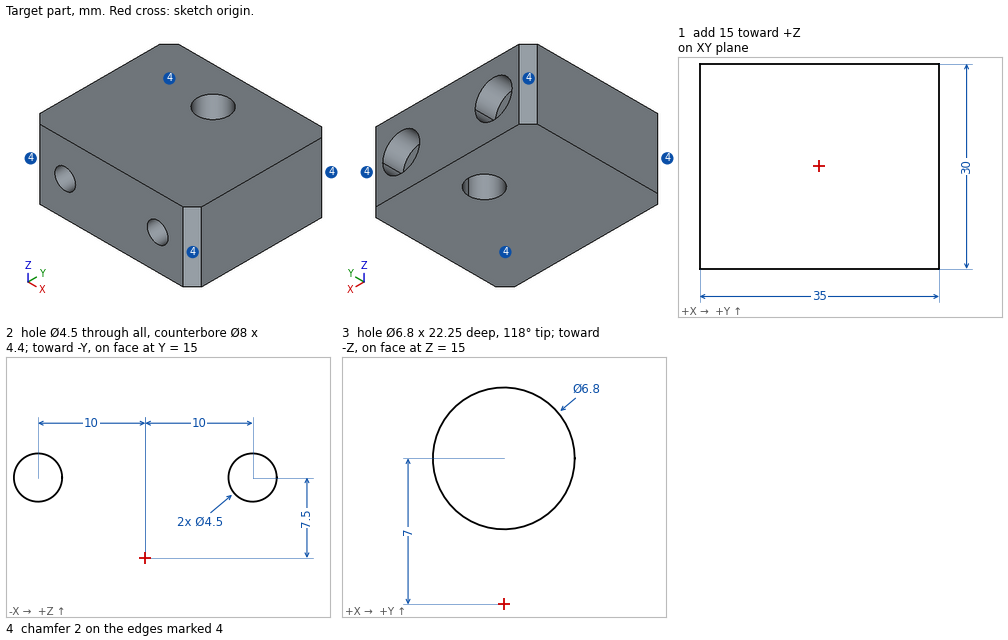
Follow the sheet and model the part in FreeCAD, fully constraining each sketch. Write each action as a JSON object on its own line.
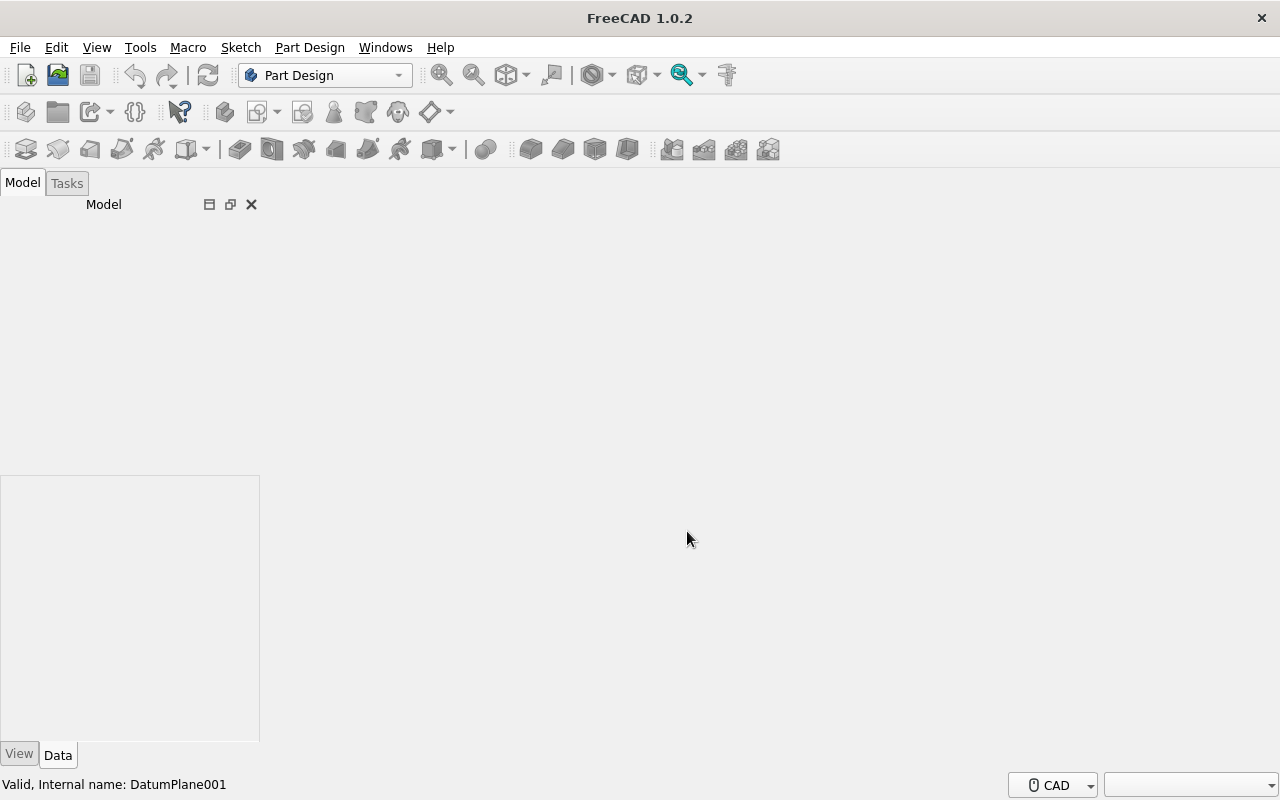
{"action": "key", "text": "ctrl+n"}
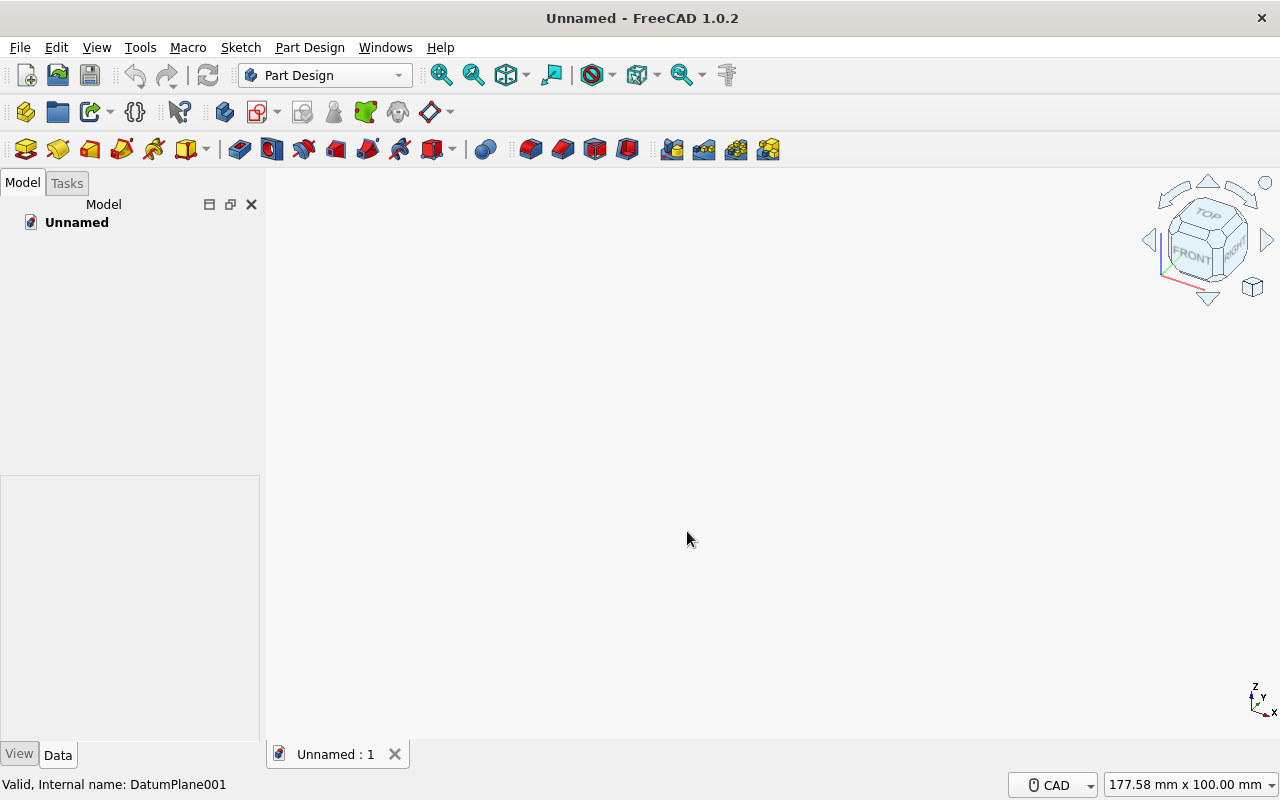
{"action": "left_click", "coordinate": [258, 112]}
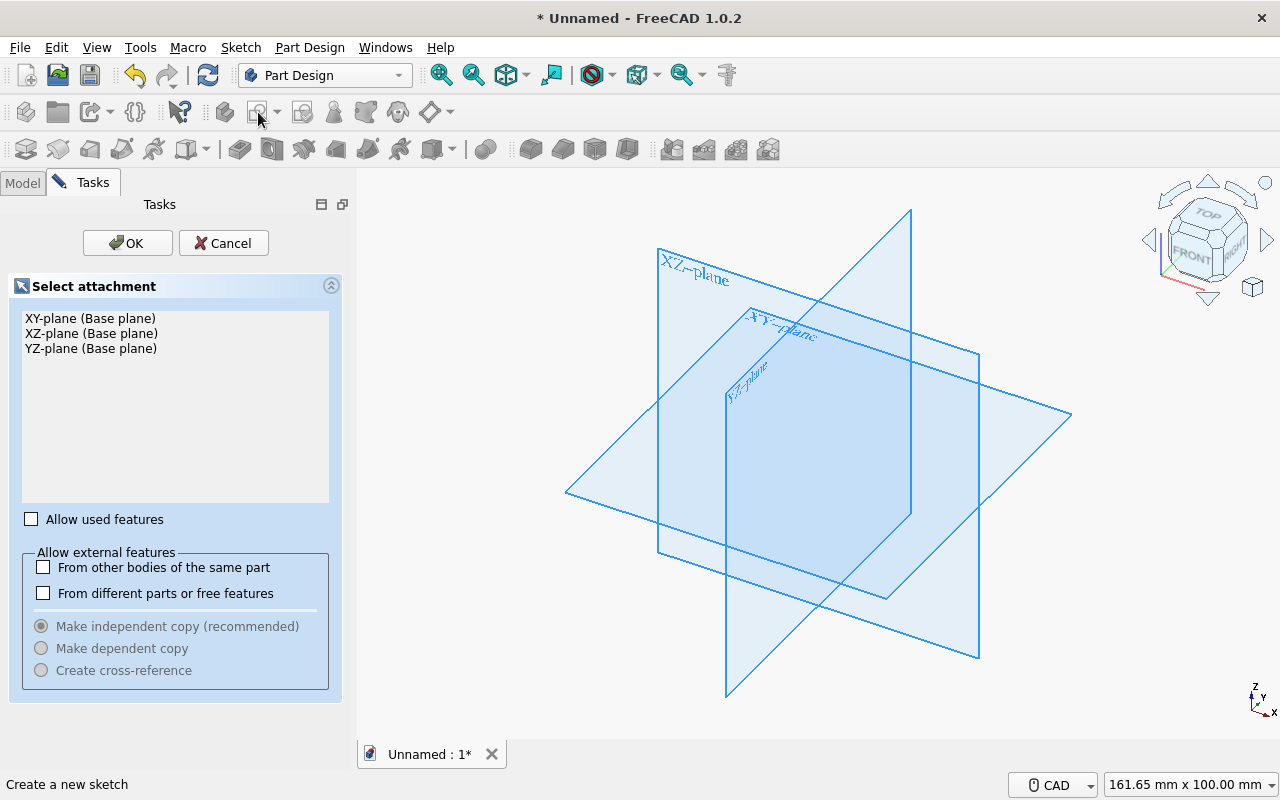
{"action": "left_click", "coordinate": [82, 318]}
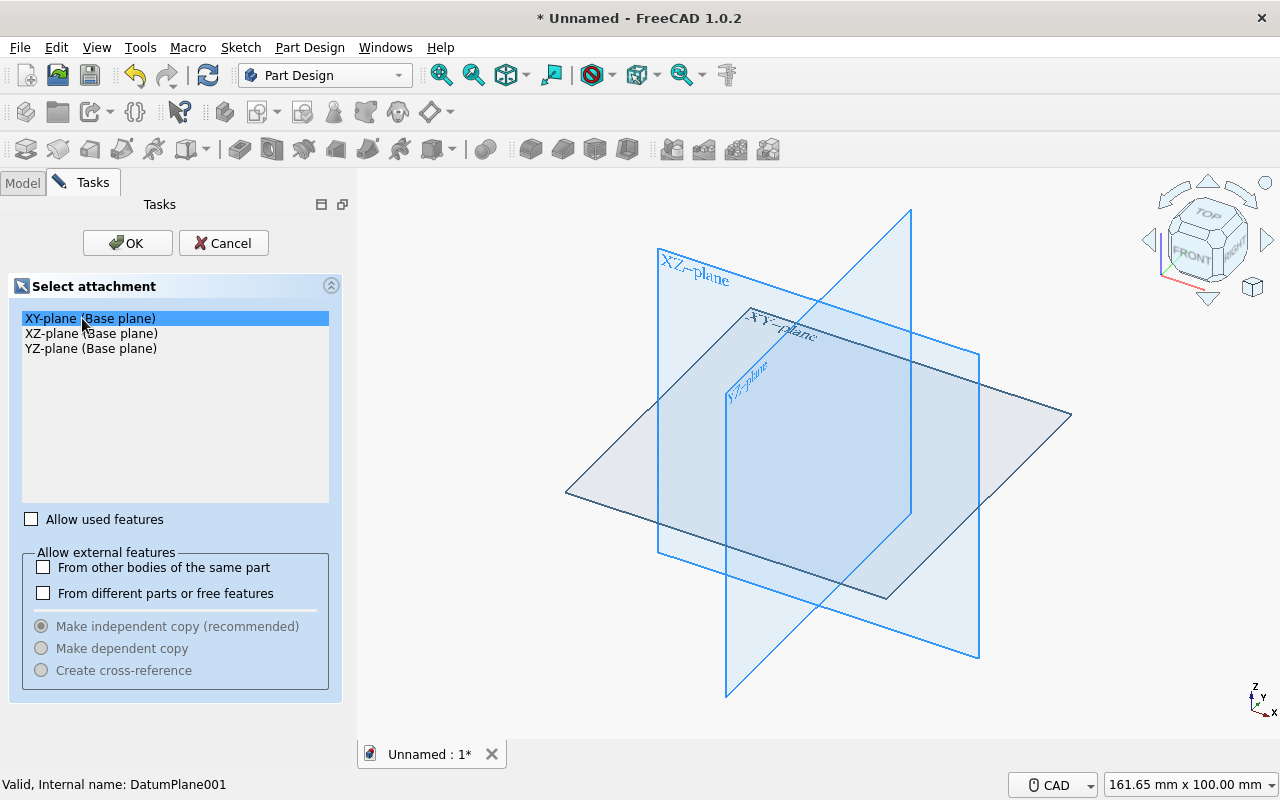
{"action": "left_click", "coordinate": [128, 243]}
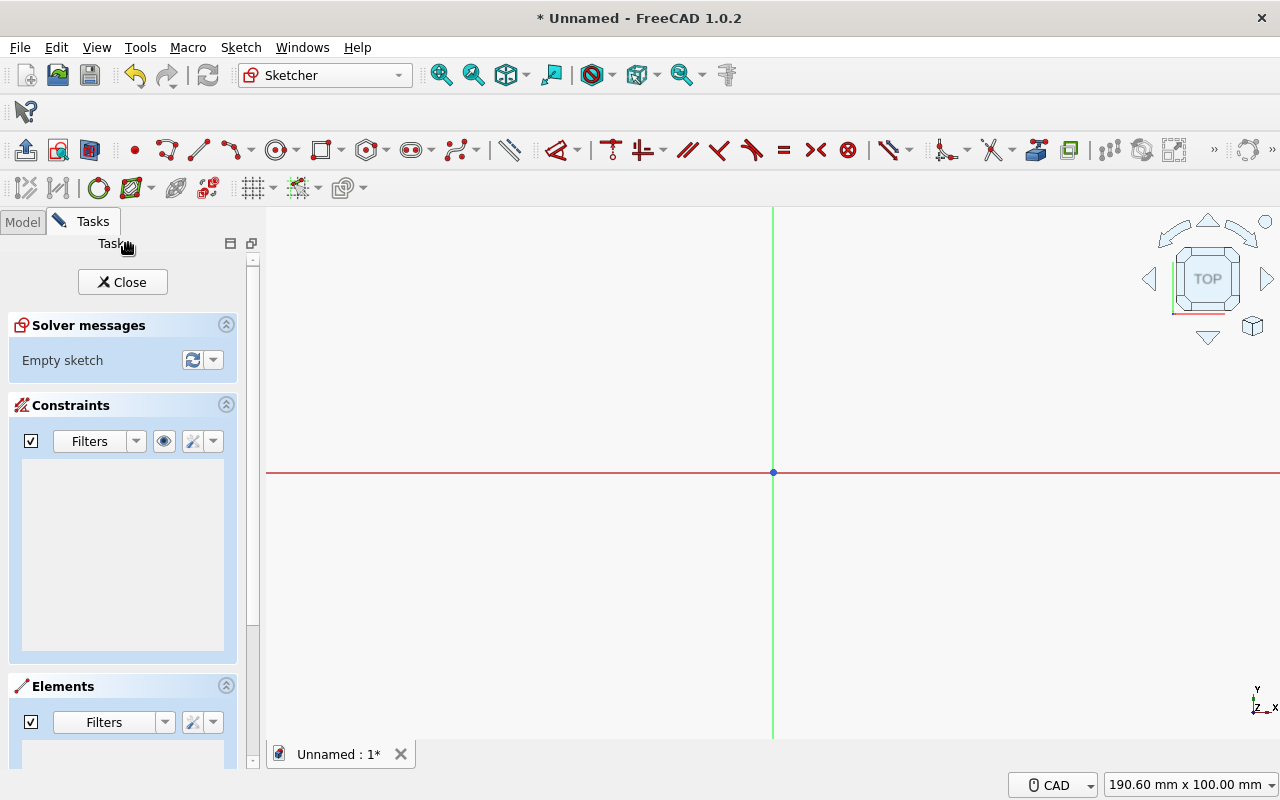
{"action": "scroll", "coordinate": [829, 473], "scroll_direction": "up", "scroll_amount": 4}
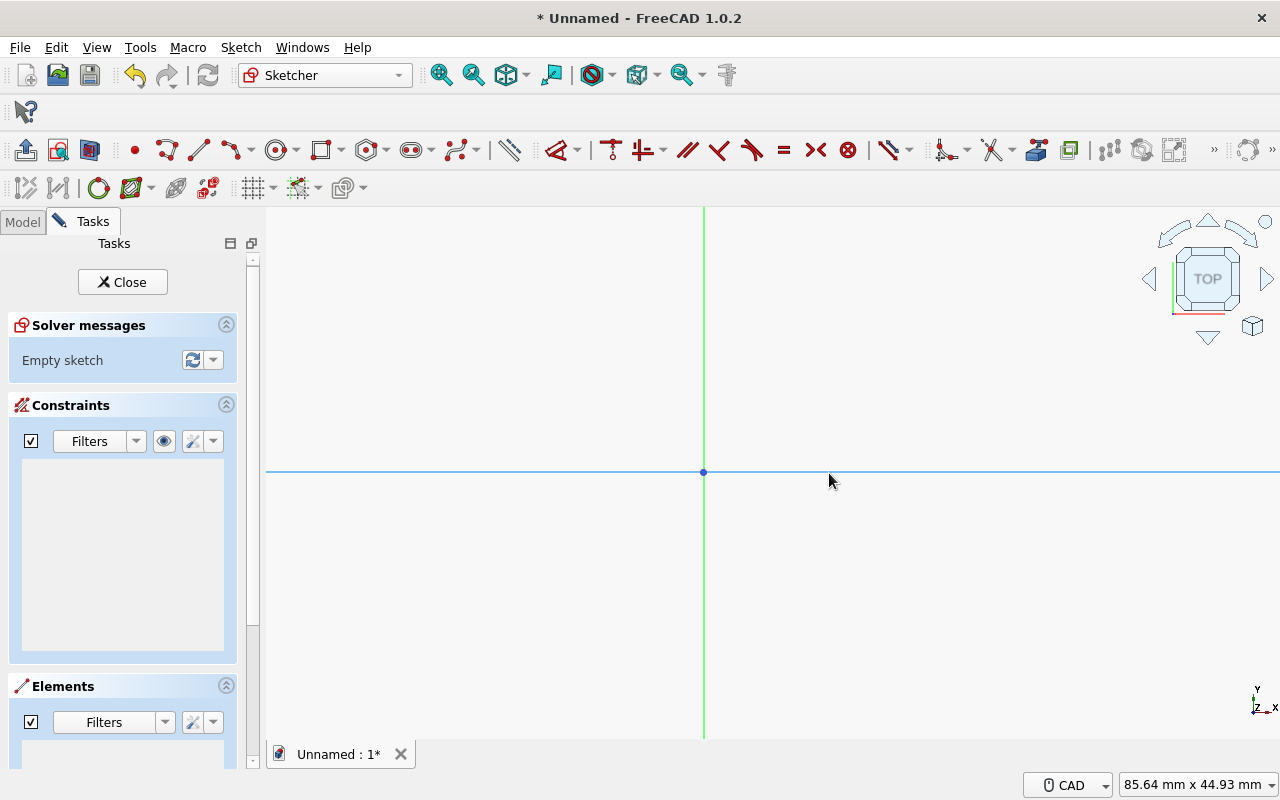
{"action": "key", "text": "g v"}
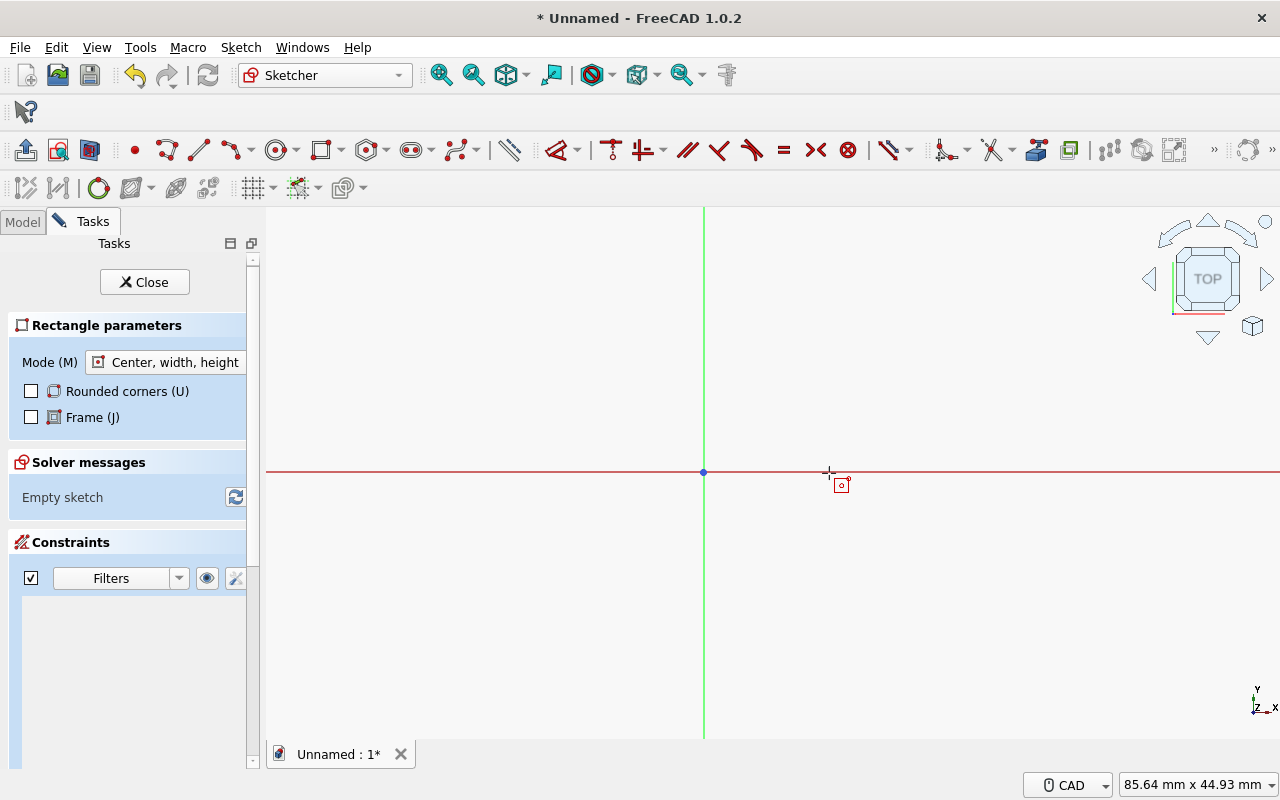
{"action": "left_click", "coordinate": [704, 472]}
{"action": "mouse_move", "coordinate": [911, 295]}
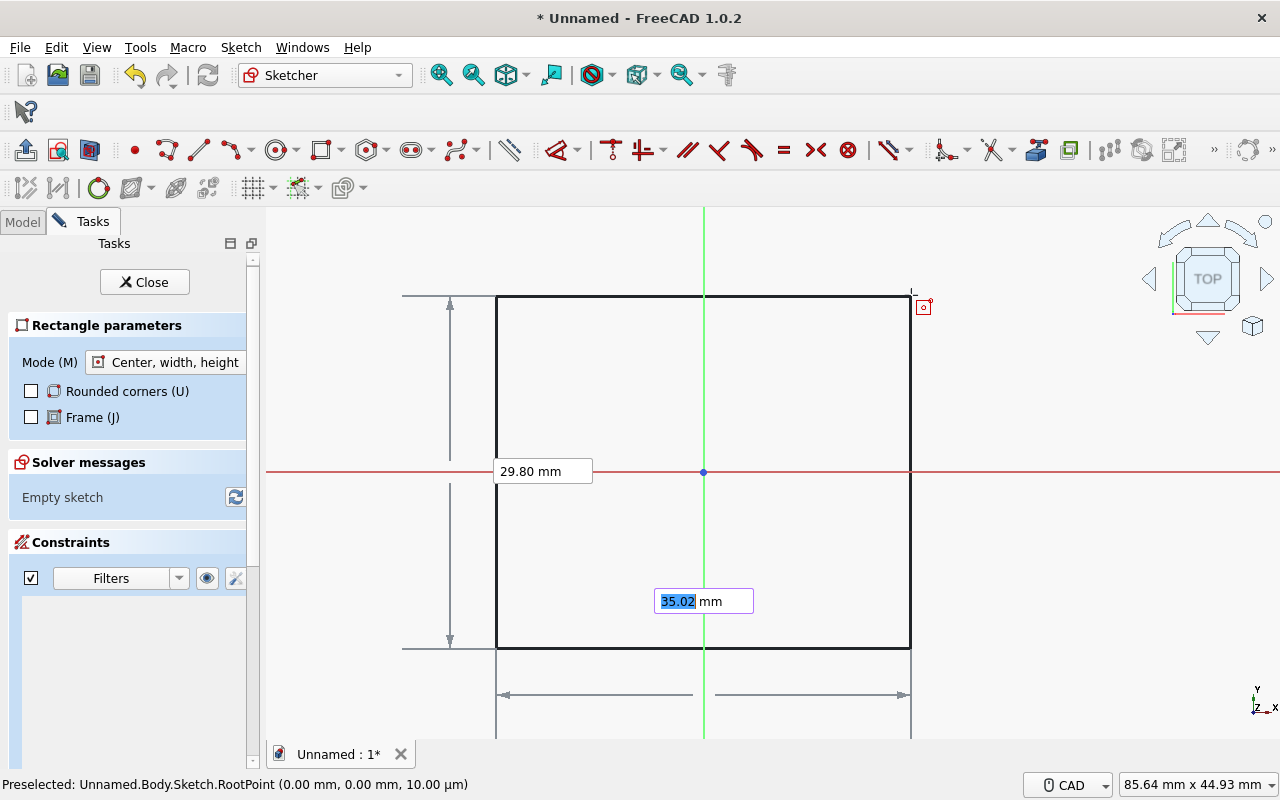
{"action": "type", "text": "35"}
{"action": "key", "text": "Tab"}
{"action": "type", "text": "30"}
{"action": "key", "text": "Return"}
{"action": "key", "text": "Escape"}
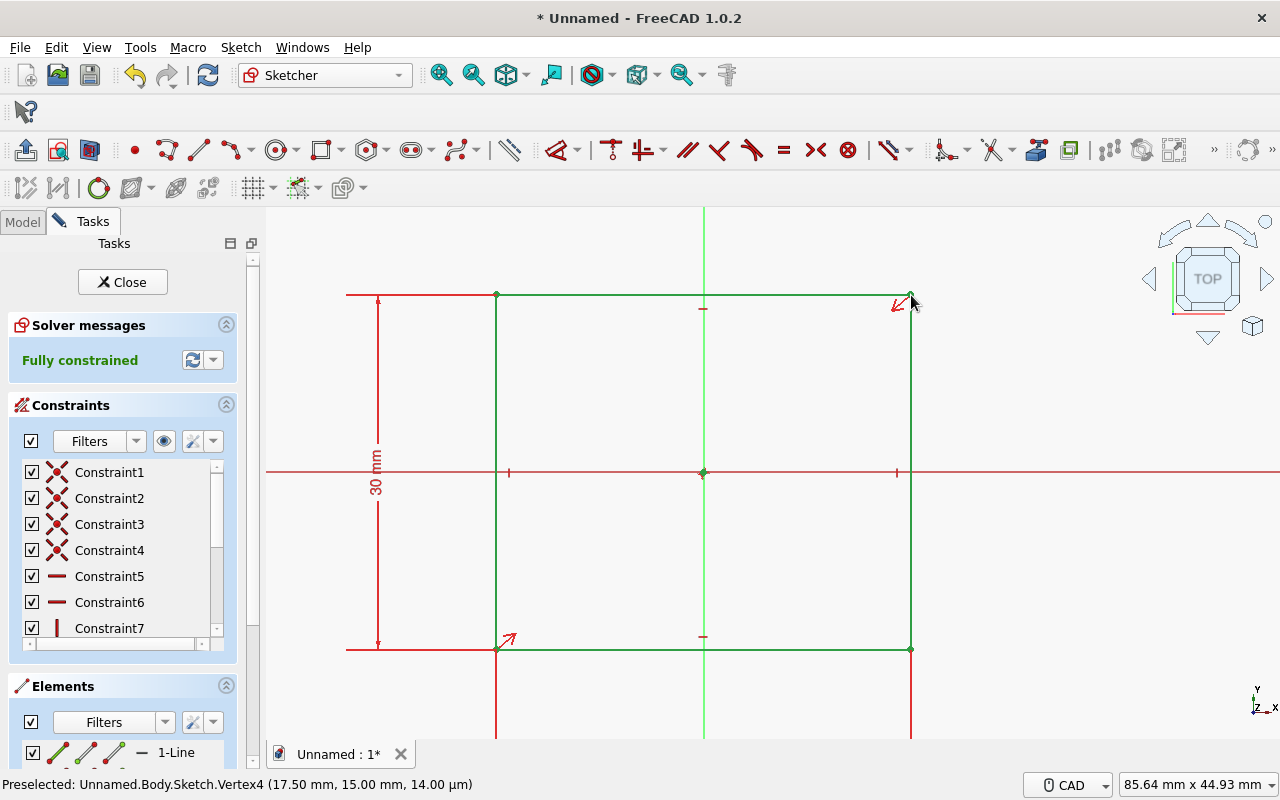
{"action": "left_click", "coordinate": [123, 282]}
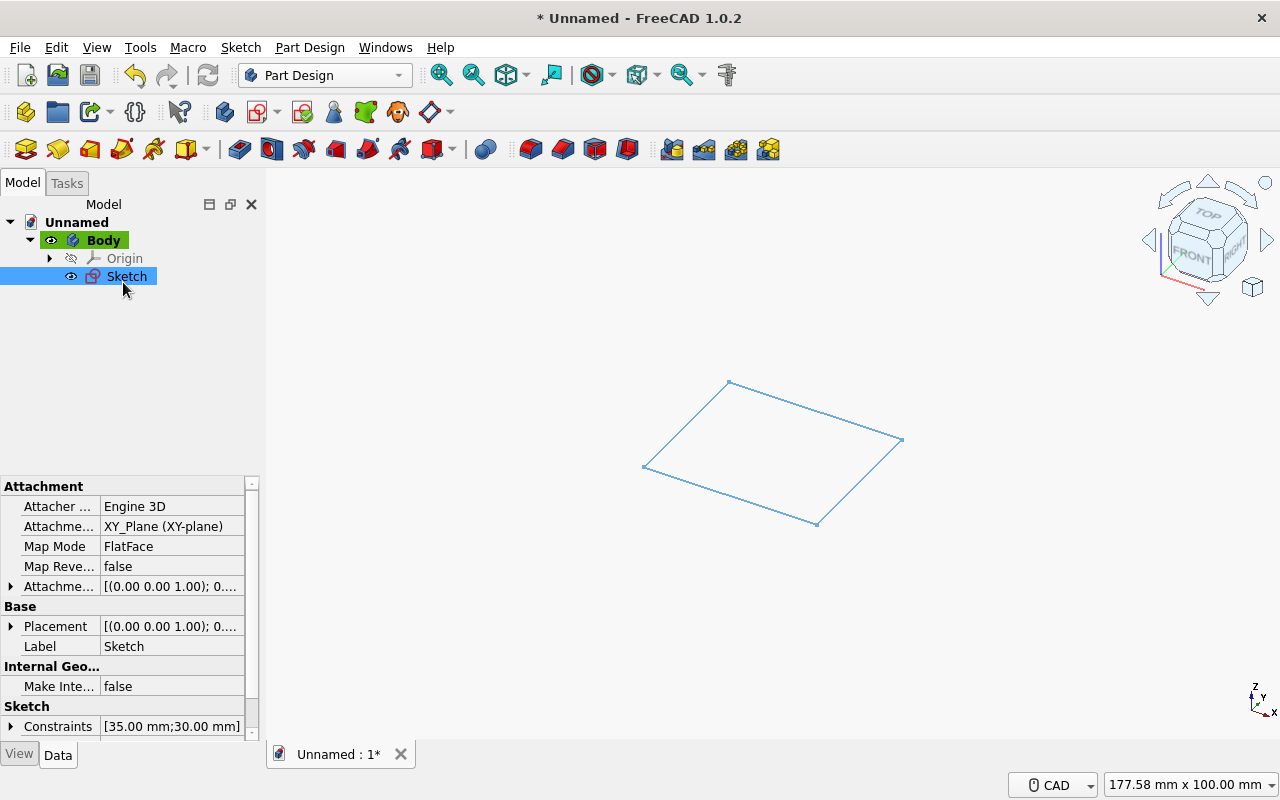
{"action": "left_click", "coordinate": [26, 150]}